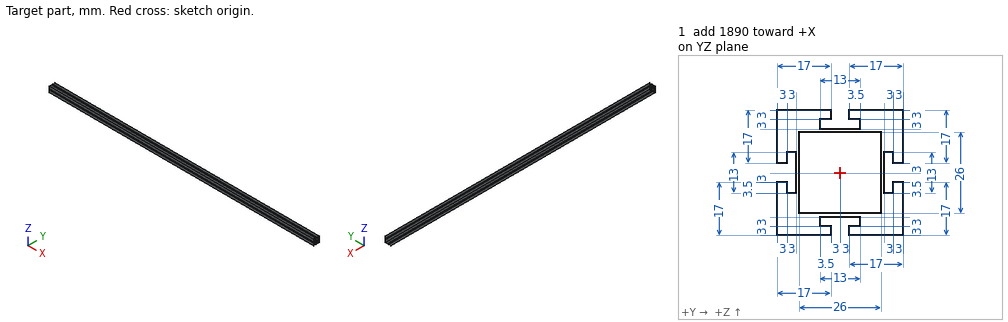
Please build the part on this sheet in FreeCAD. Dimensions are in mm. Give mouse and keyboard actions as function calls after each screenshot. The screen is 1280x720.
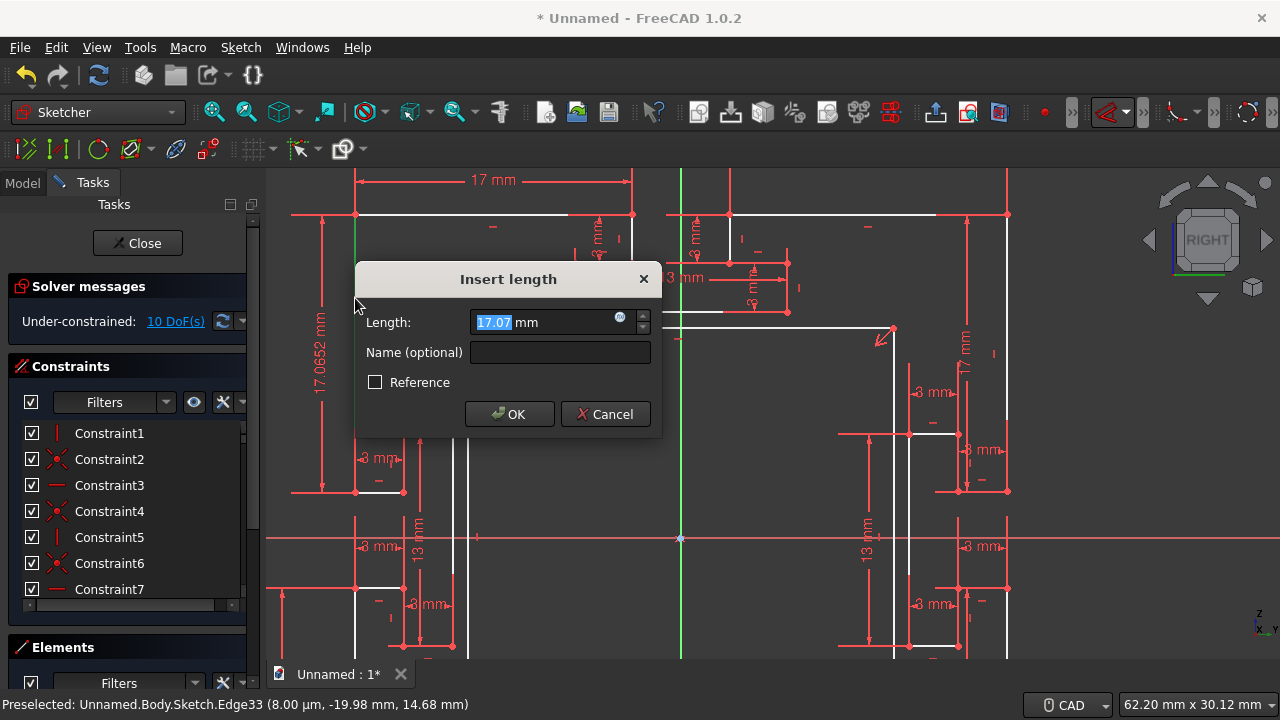
text(17)
key(Return)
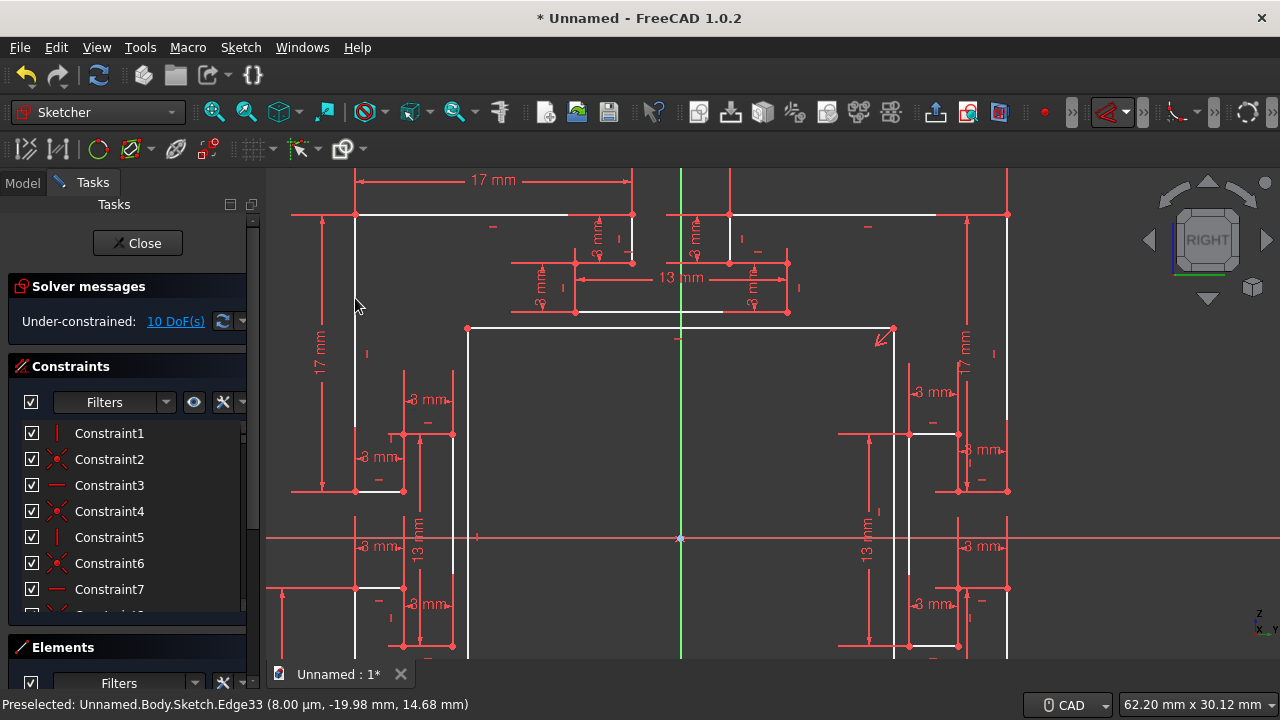
scroll(724, 312, down, 4)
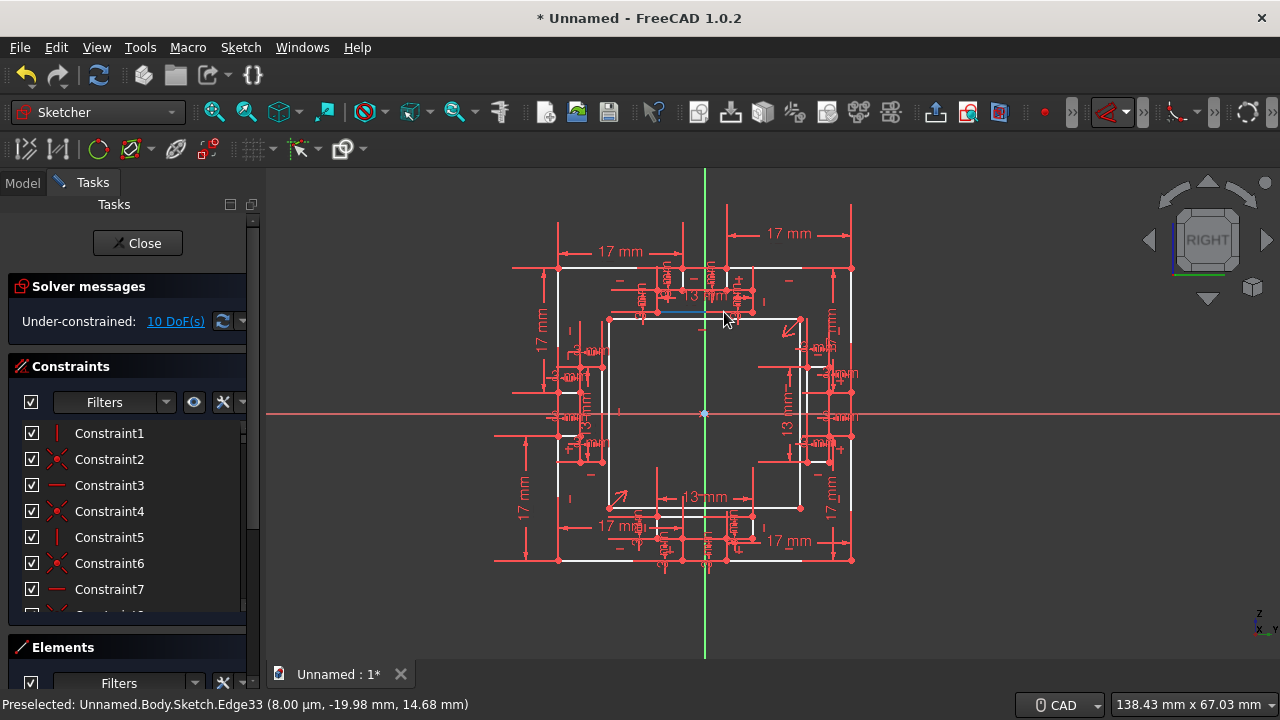
scroll(667, 508, up, 3)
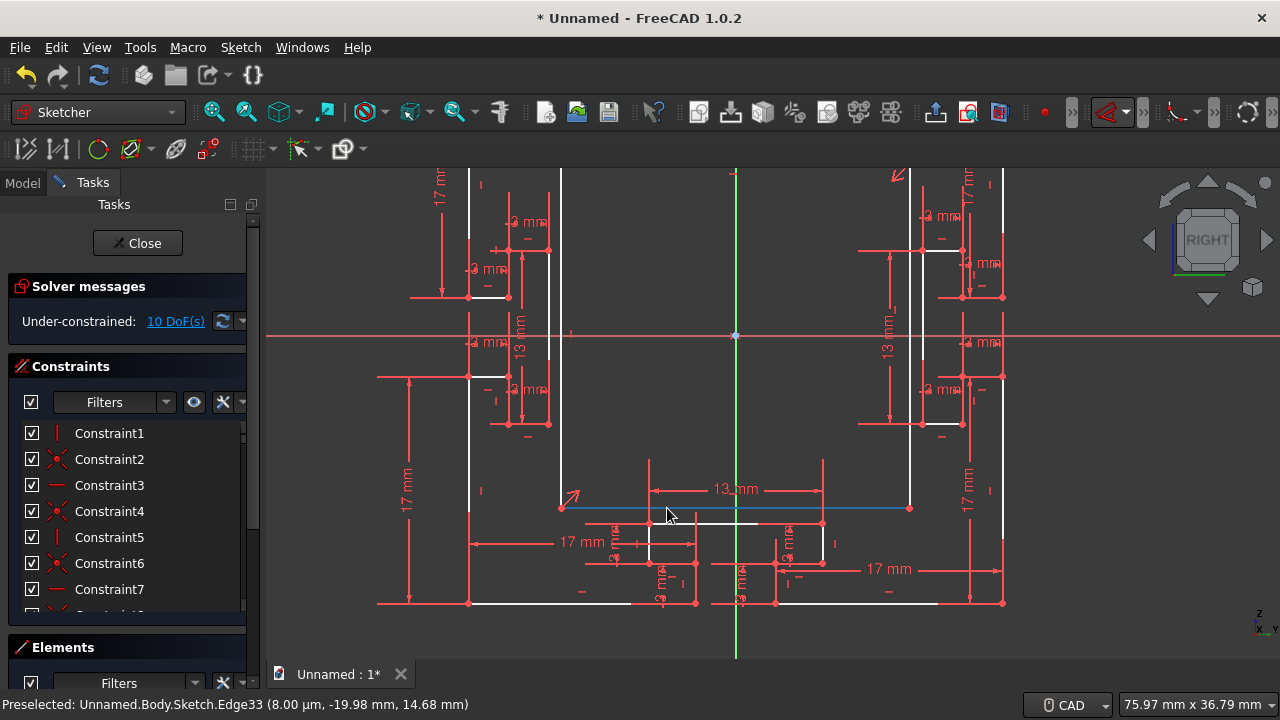
click(666, 508)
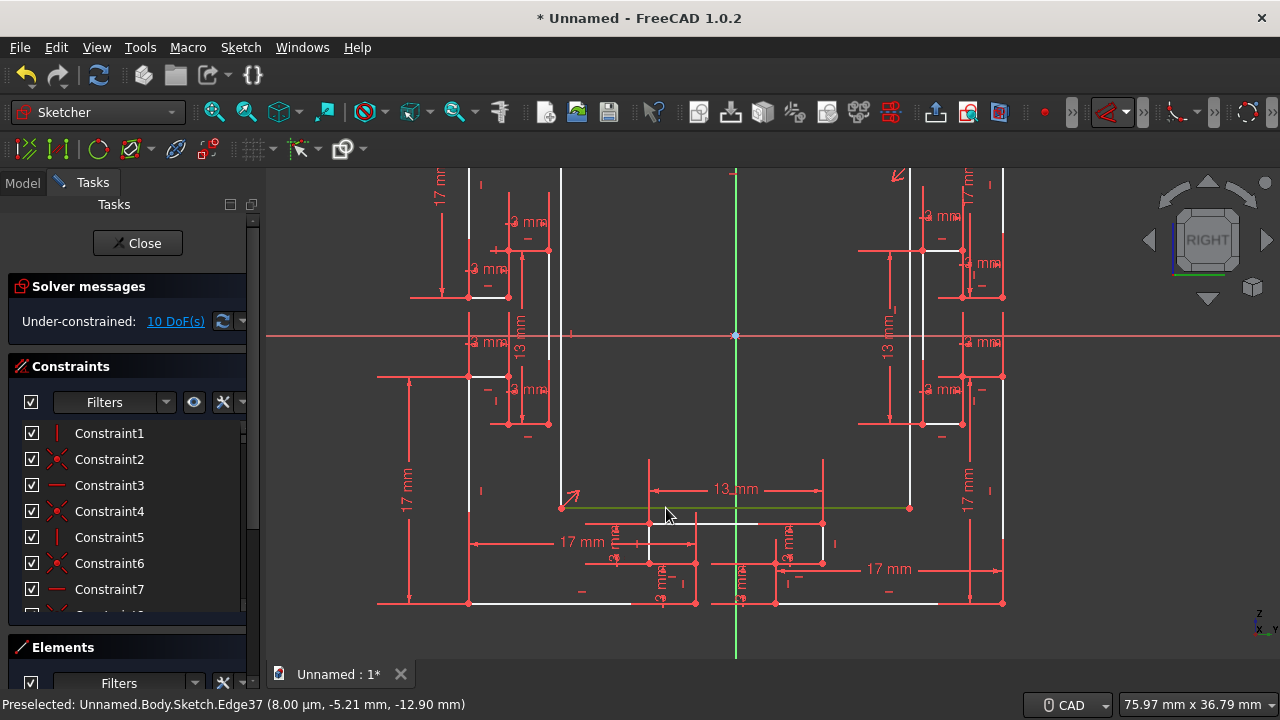
click(1128, 112)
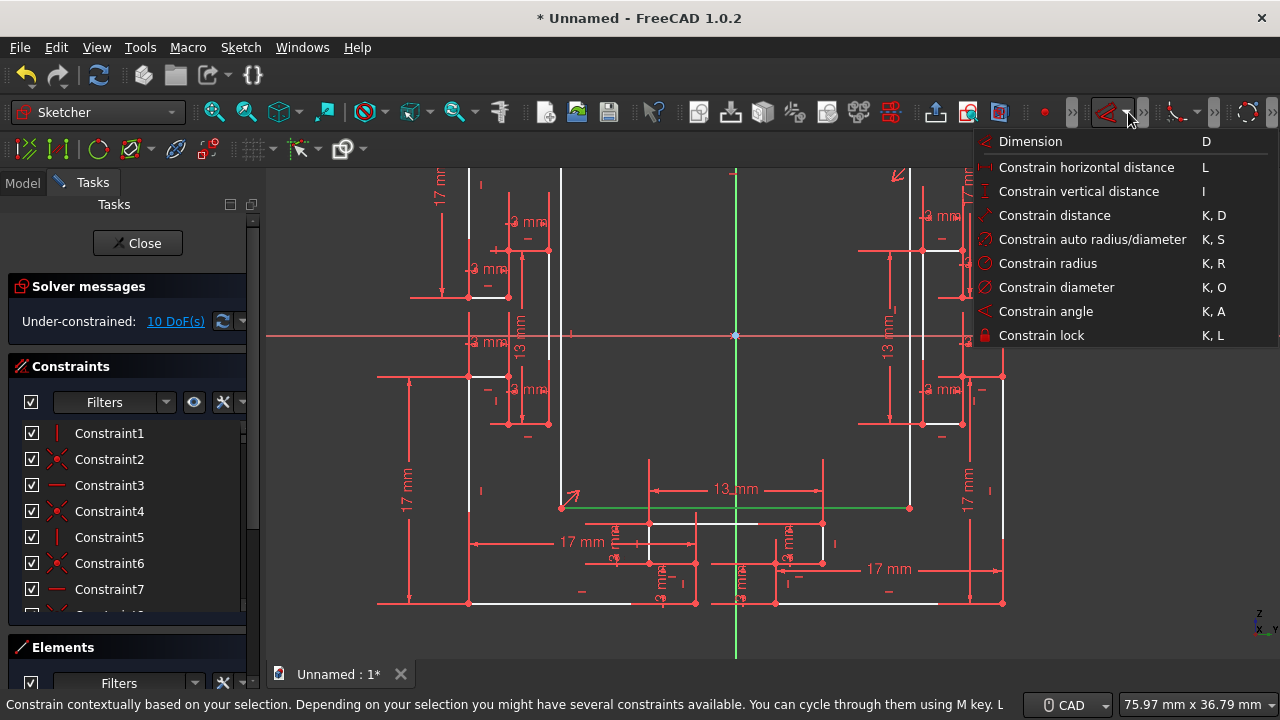
click(1126, 167)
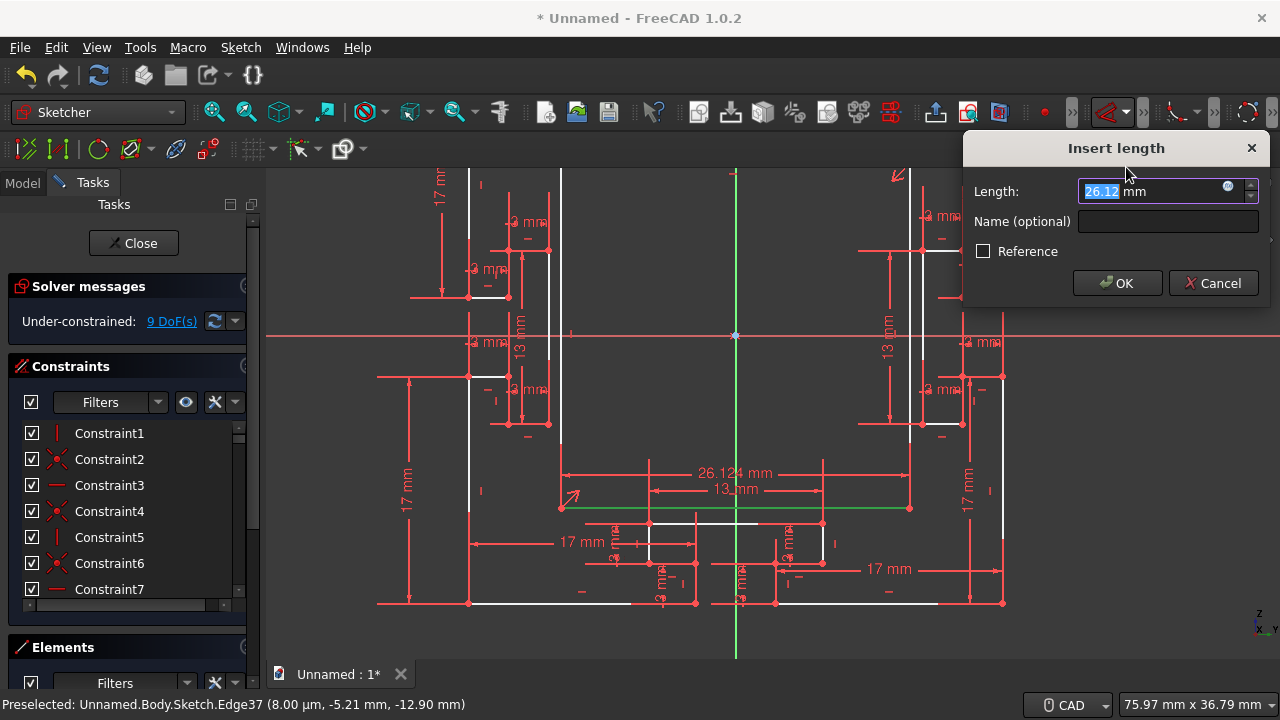
text(26)
key(Return)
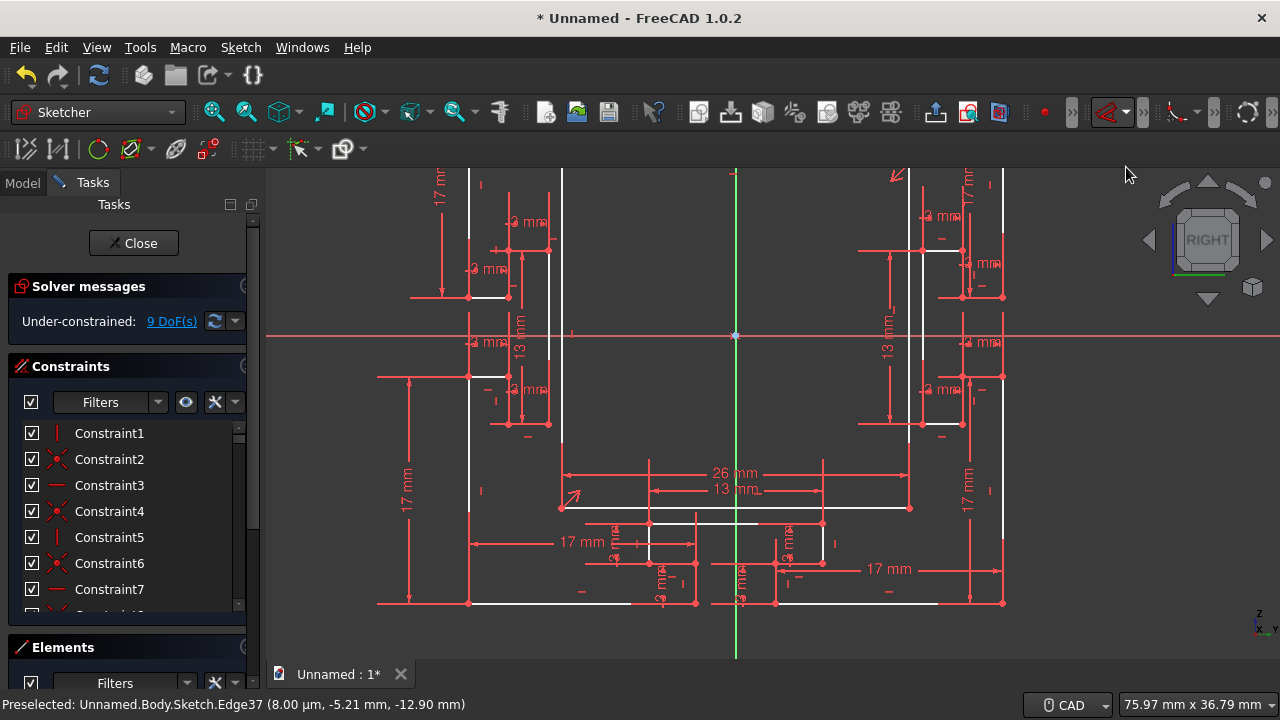
click(909, 405)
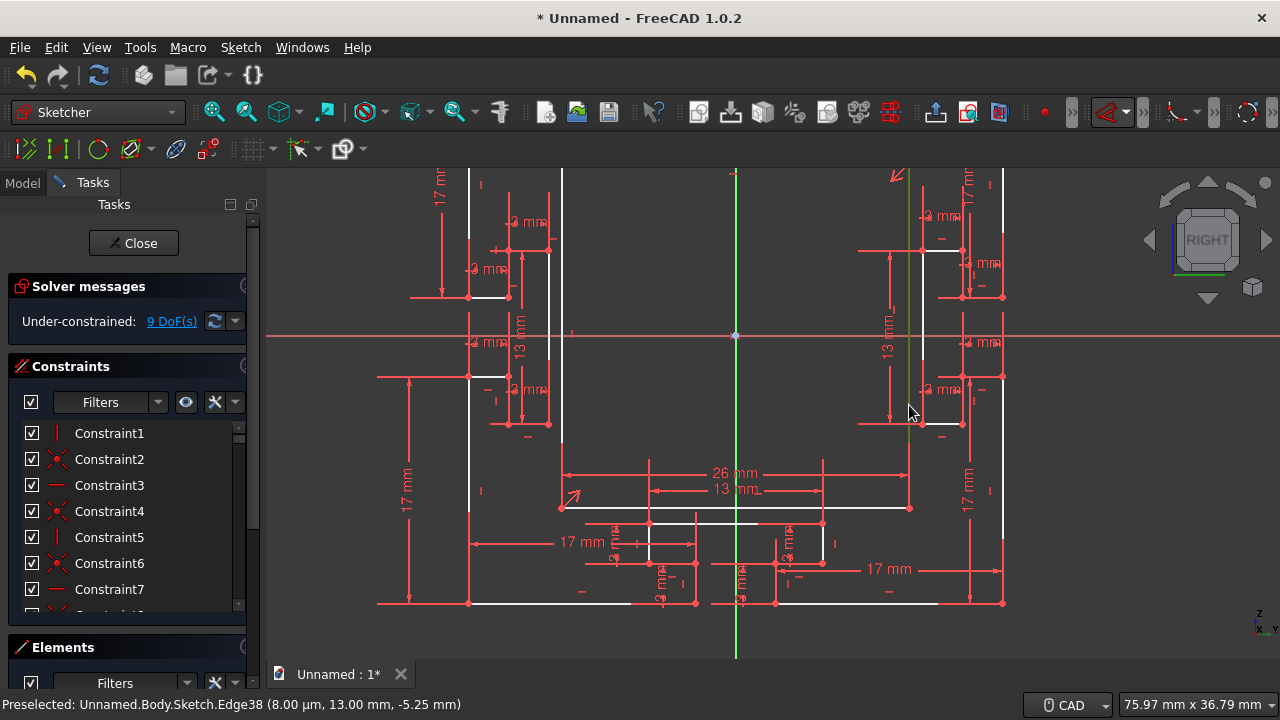
key(i)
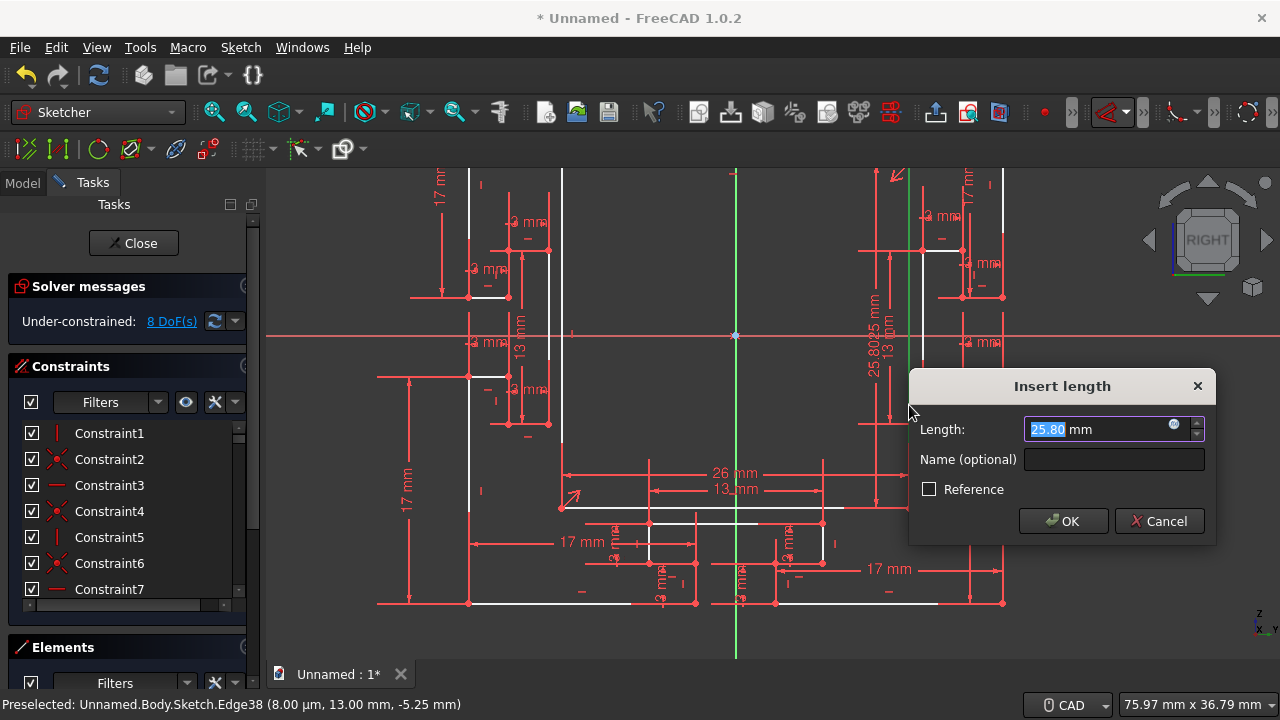
text(26)
key(Return)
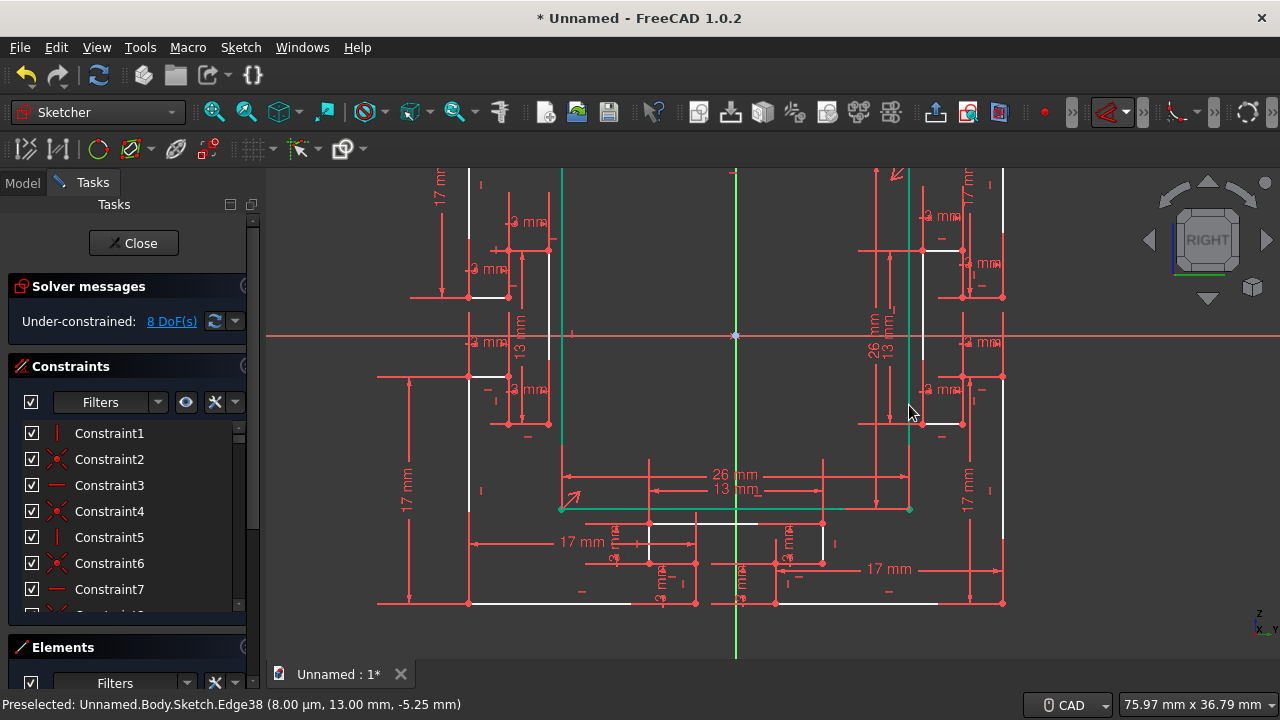
click(509, 377)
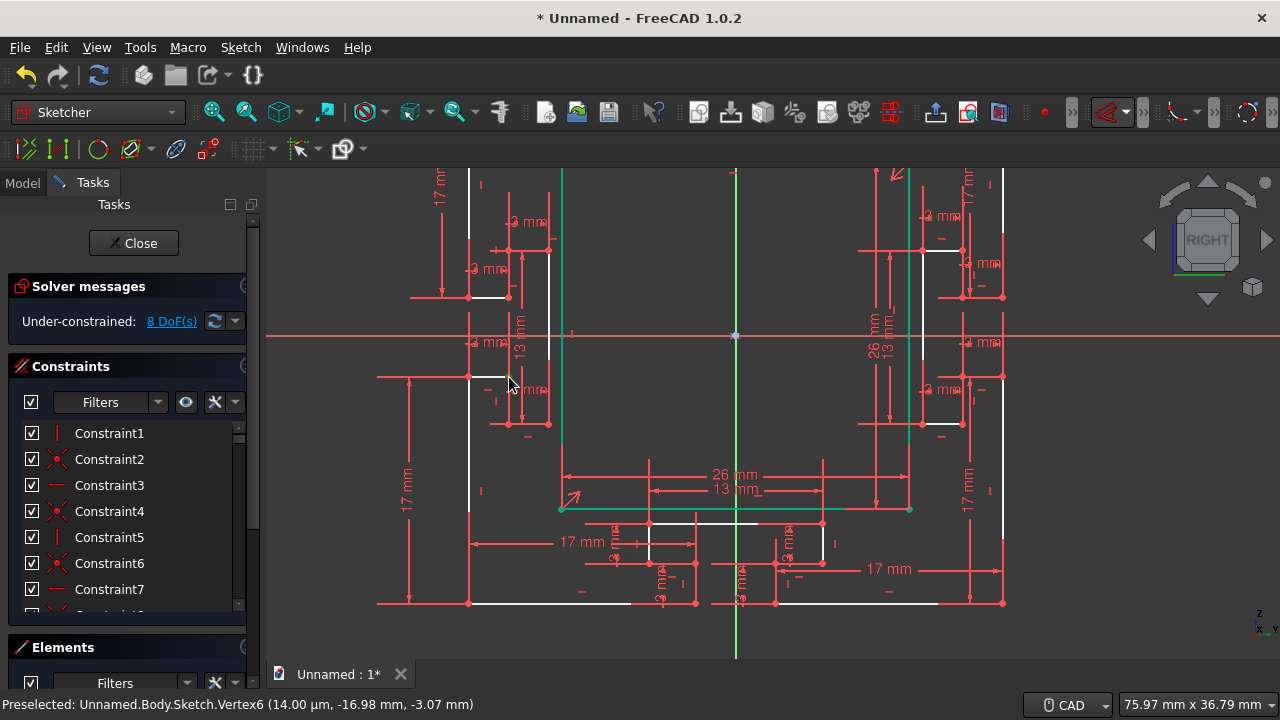
key(i)